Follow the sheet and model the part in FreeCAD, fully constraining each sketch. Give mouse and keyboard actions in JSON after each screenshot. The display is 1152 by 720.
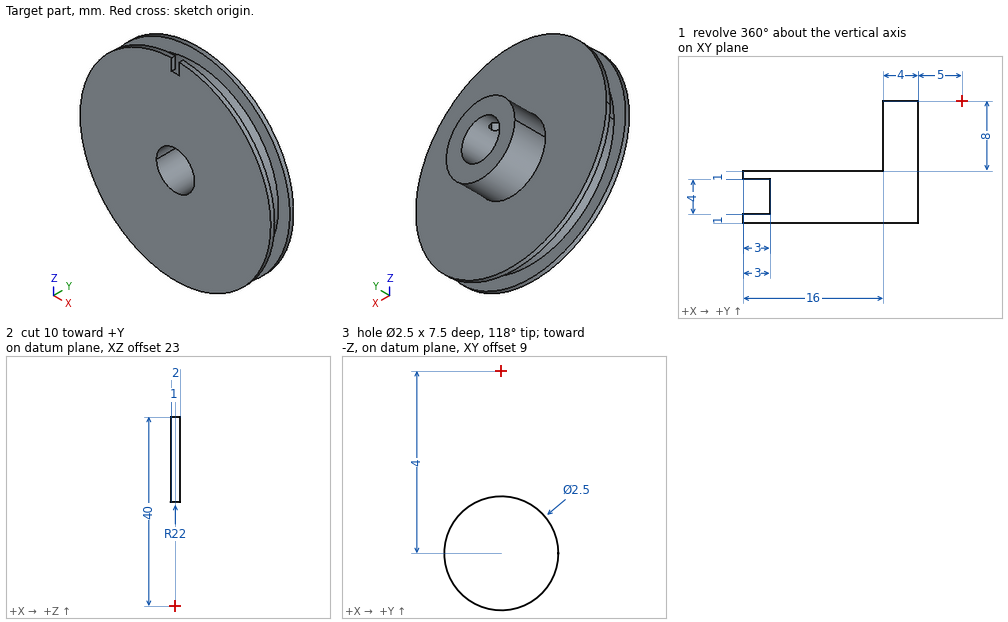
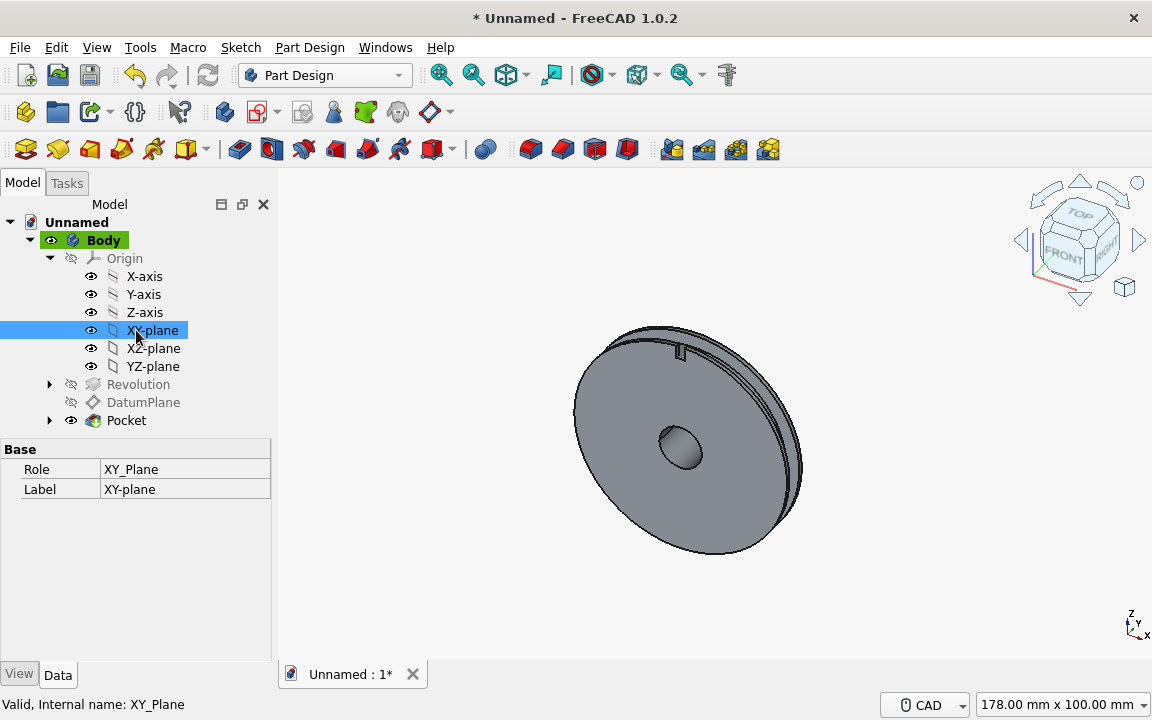
{"action": "left_click", "coordinate": [430, 112]}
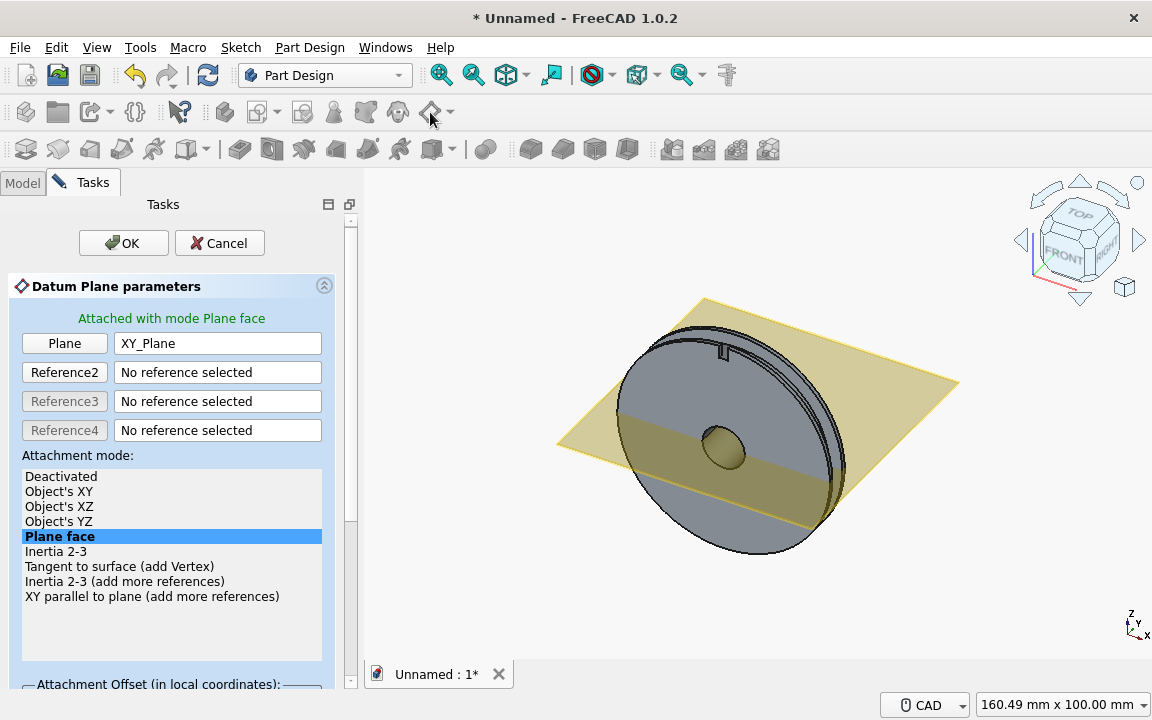
{"action": "scroll", "coordinate": [351, 451], "scroll_direction": "down", "scroll_amount": 3}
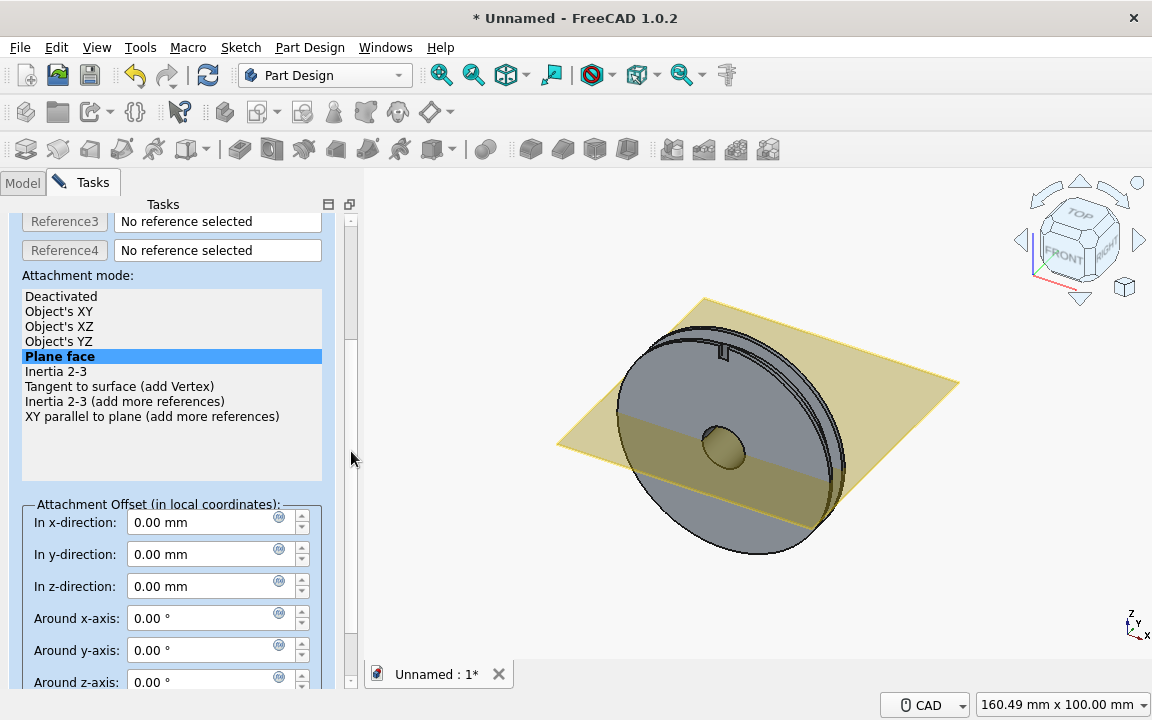
{"action": "triple_click", "coordinate": [210, 586]}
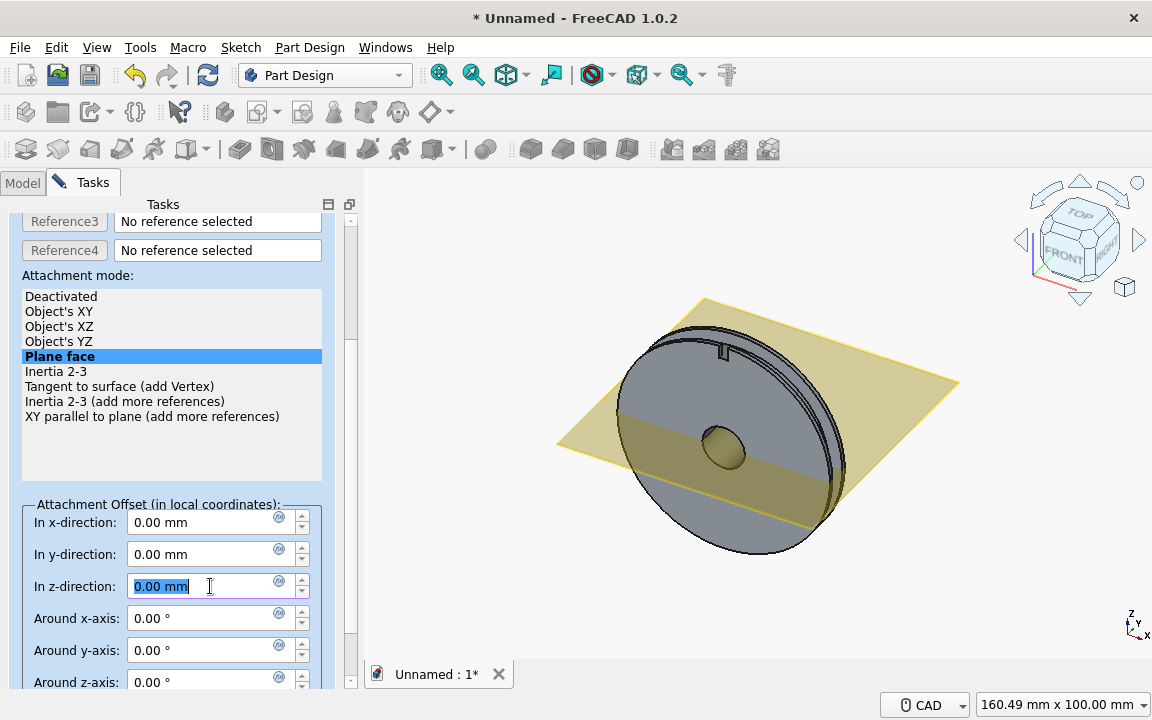
{"action": "type", "text": "9"}
{"action": "key", "text": "Tab"}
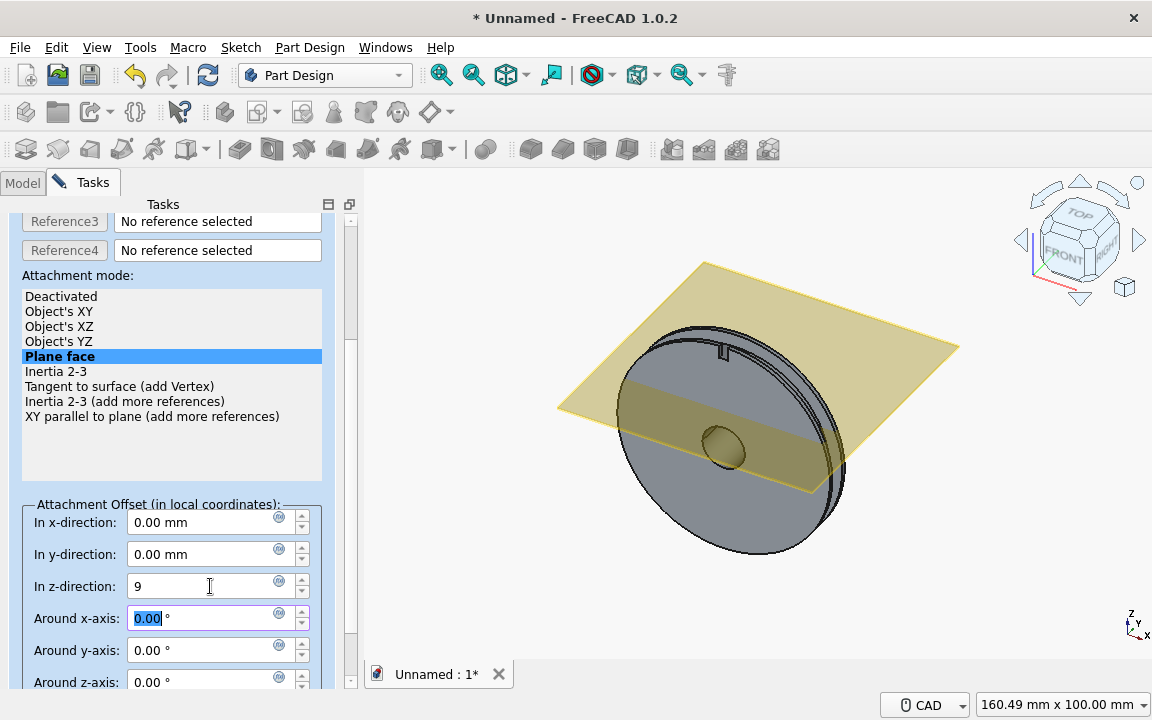
{"action": "scroll", "coordinate": [351, 451], "scroll_direction": "up", "scroll_amount": 4}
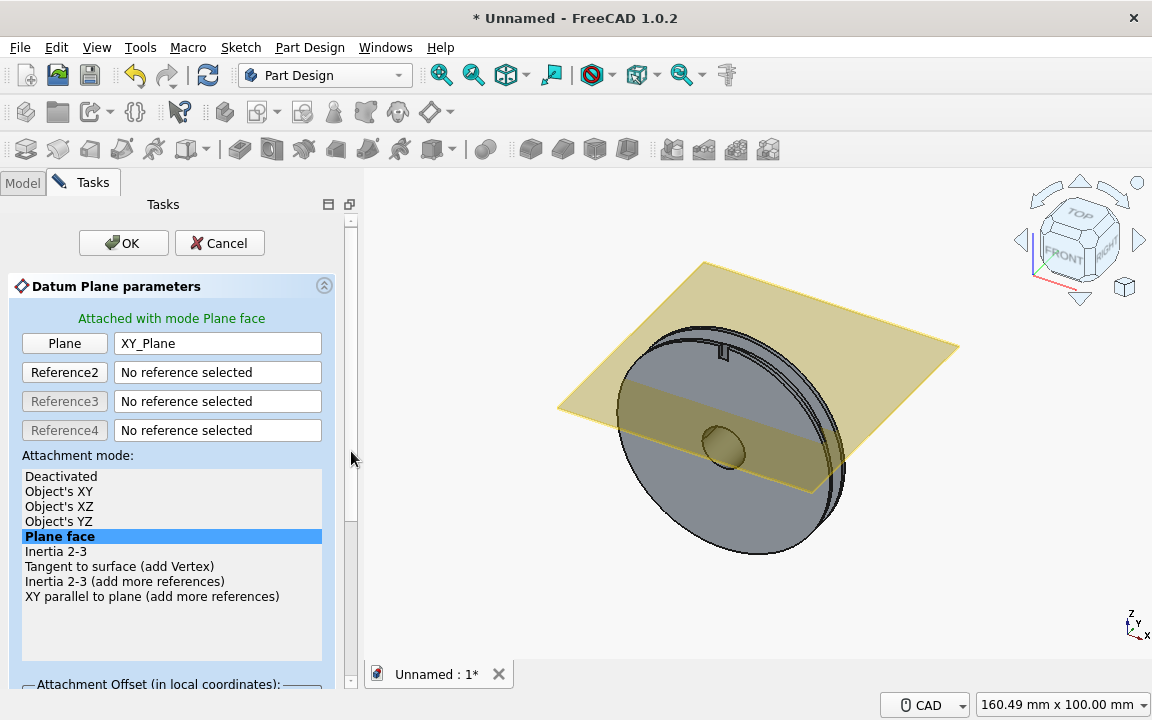
{"action": "left_click", "coordinate": [124, 243]}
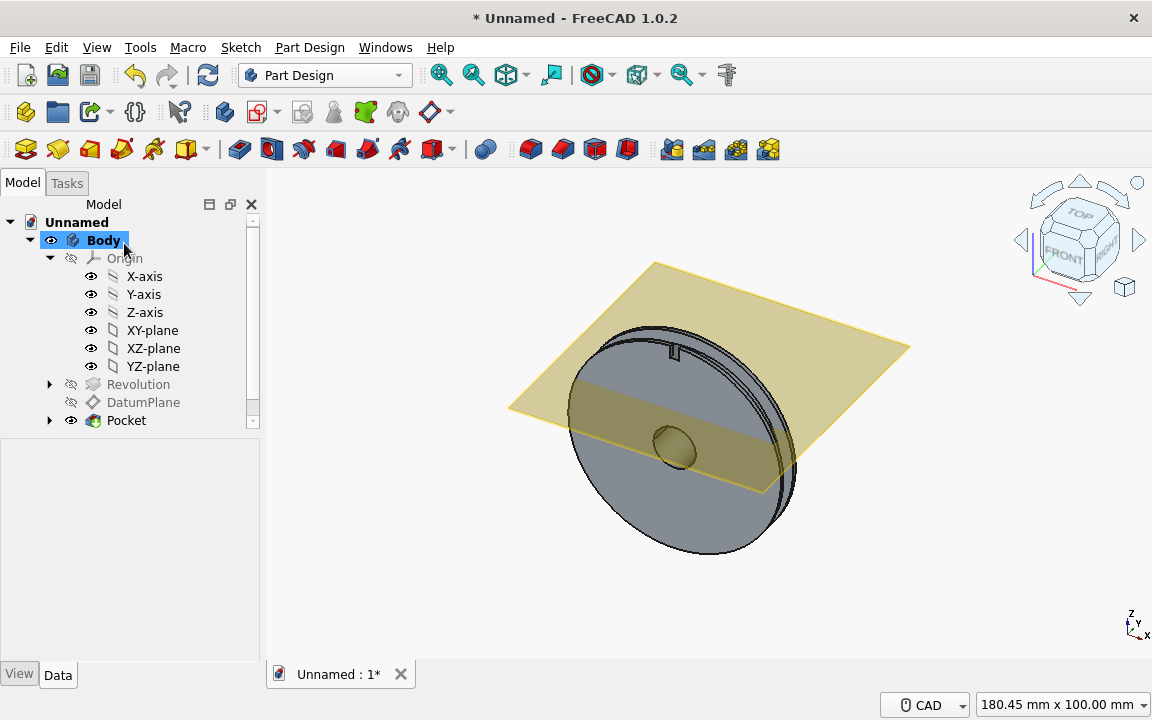
{"action": "scroll", "coordinate": [100, 326], "scroll_direction": "down", "scroll_amount": 3}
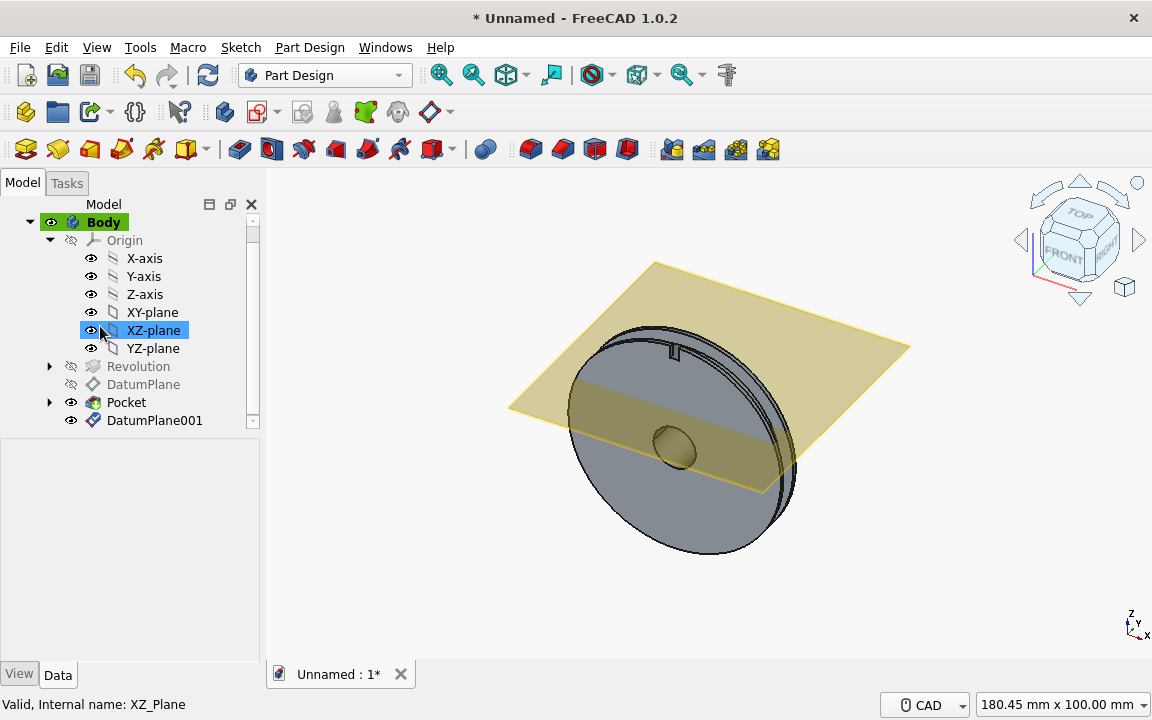
{"action": "left_click", "coordinate": [116, 420]}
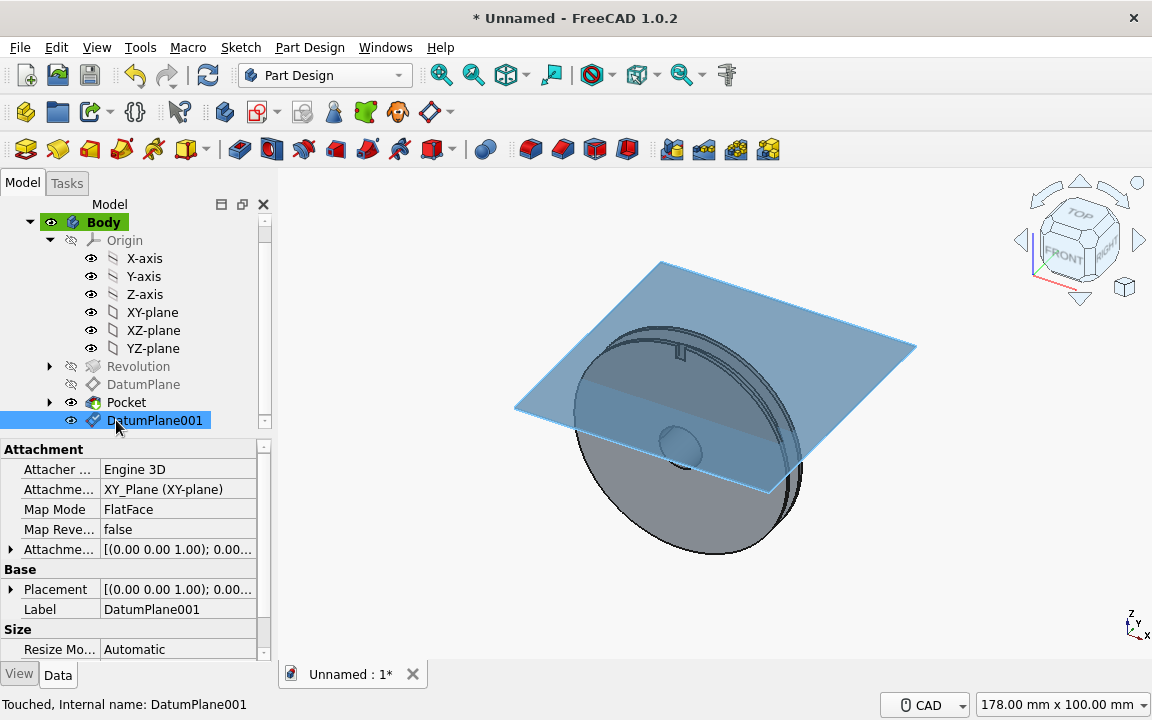
{"action": "left_click", "coordinate": [258, 112]}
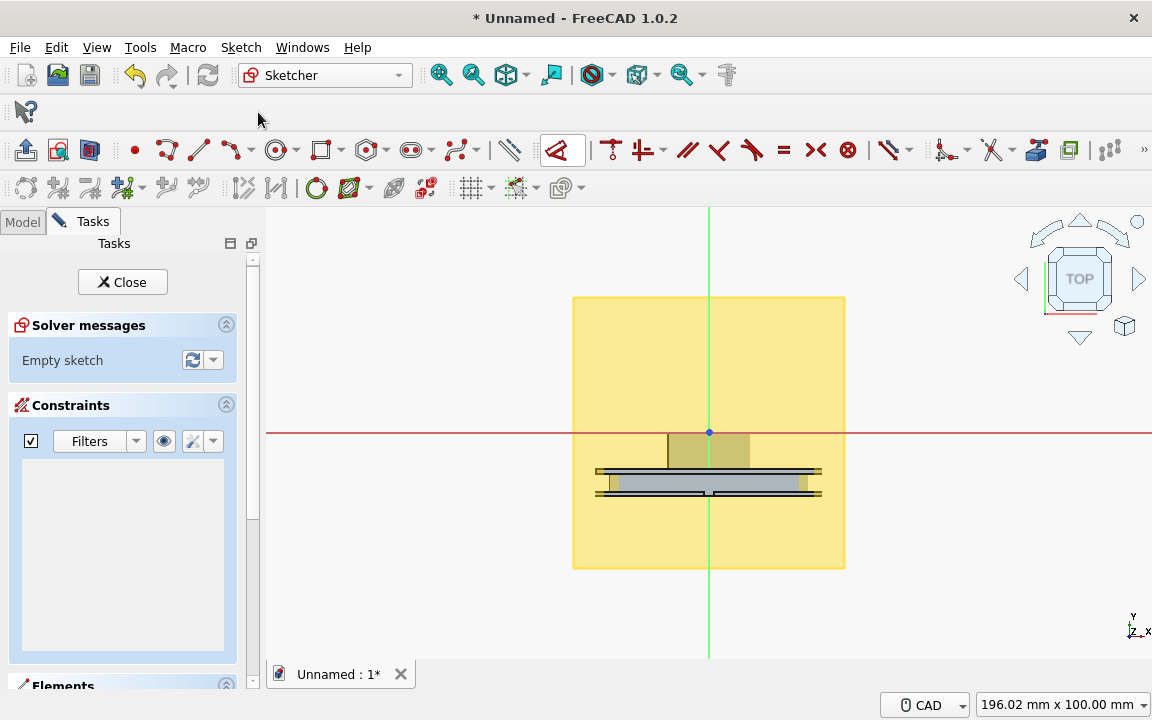
{"action": "left_click", "coordinate": [90, 150]}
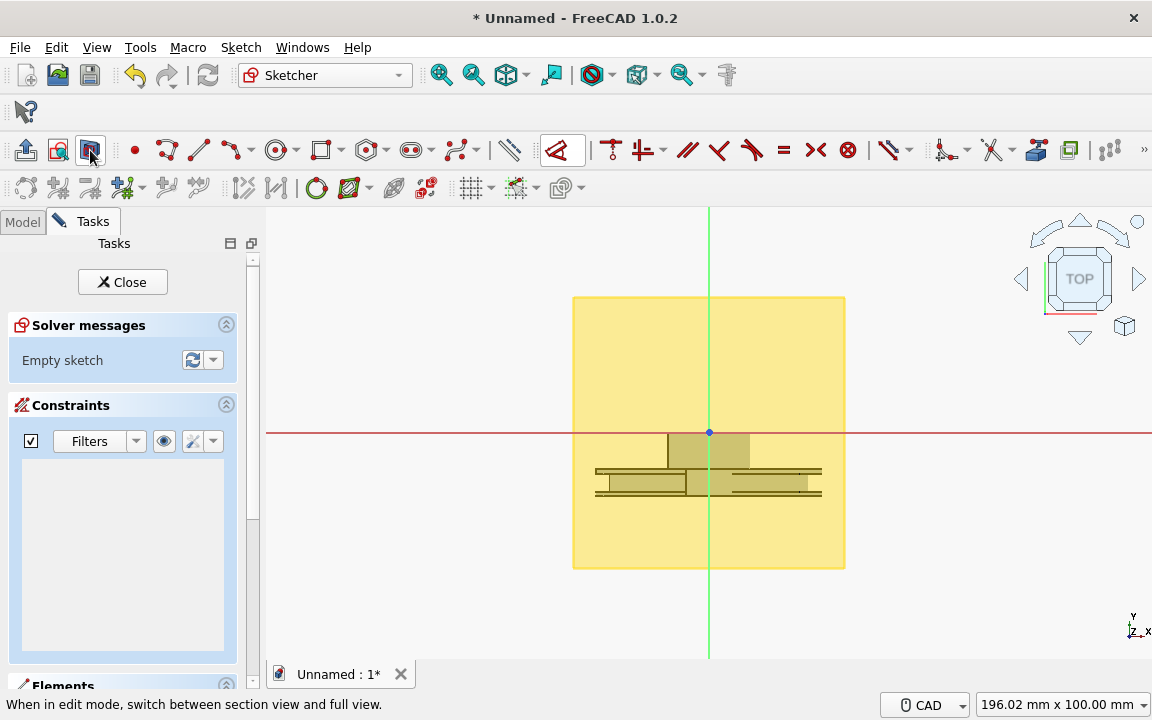
{"action": "scroll", "coordinate": [716, 446], "scroll_direction": "up", "scroll_amount": 12}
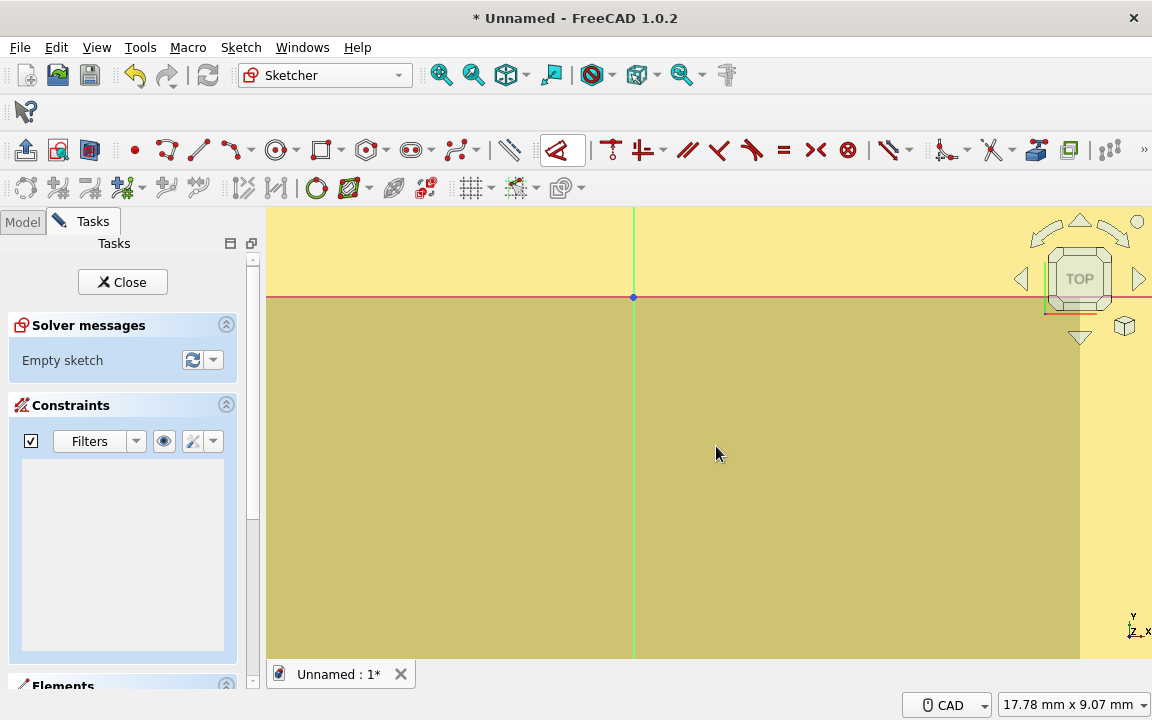
{"action": "key", "text": "g c"}